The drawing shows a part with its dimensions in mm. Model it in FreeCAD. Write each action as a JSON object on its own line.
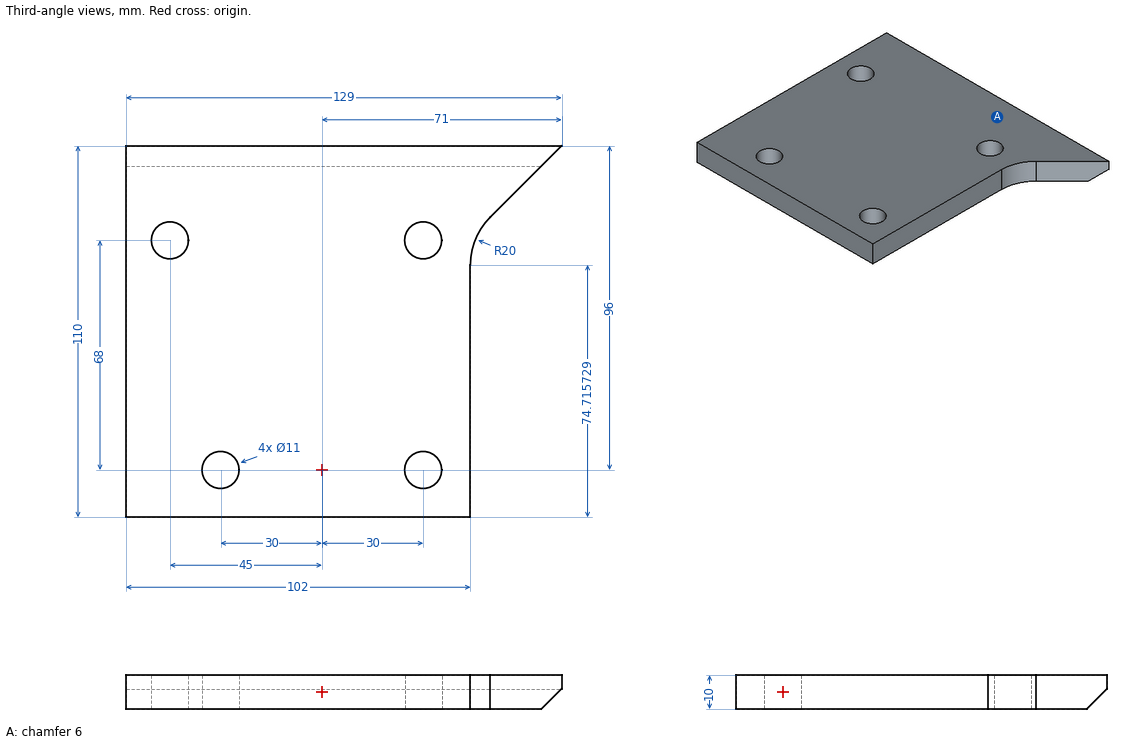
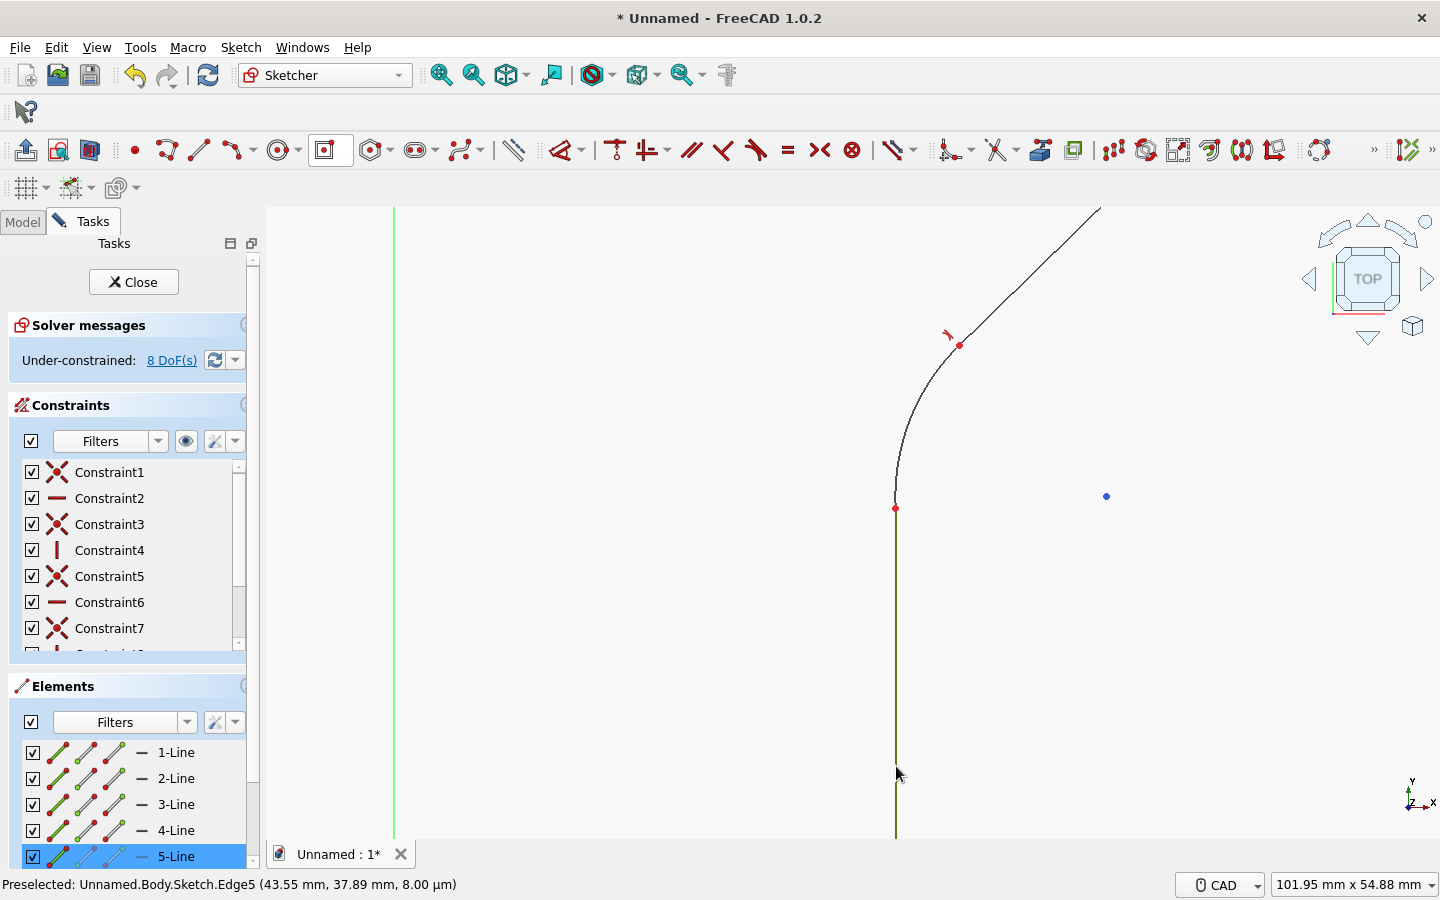
{"action": "left_click", "coordinate": [926, 388]}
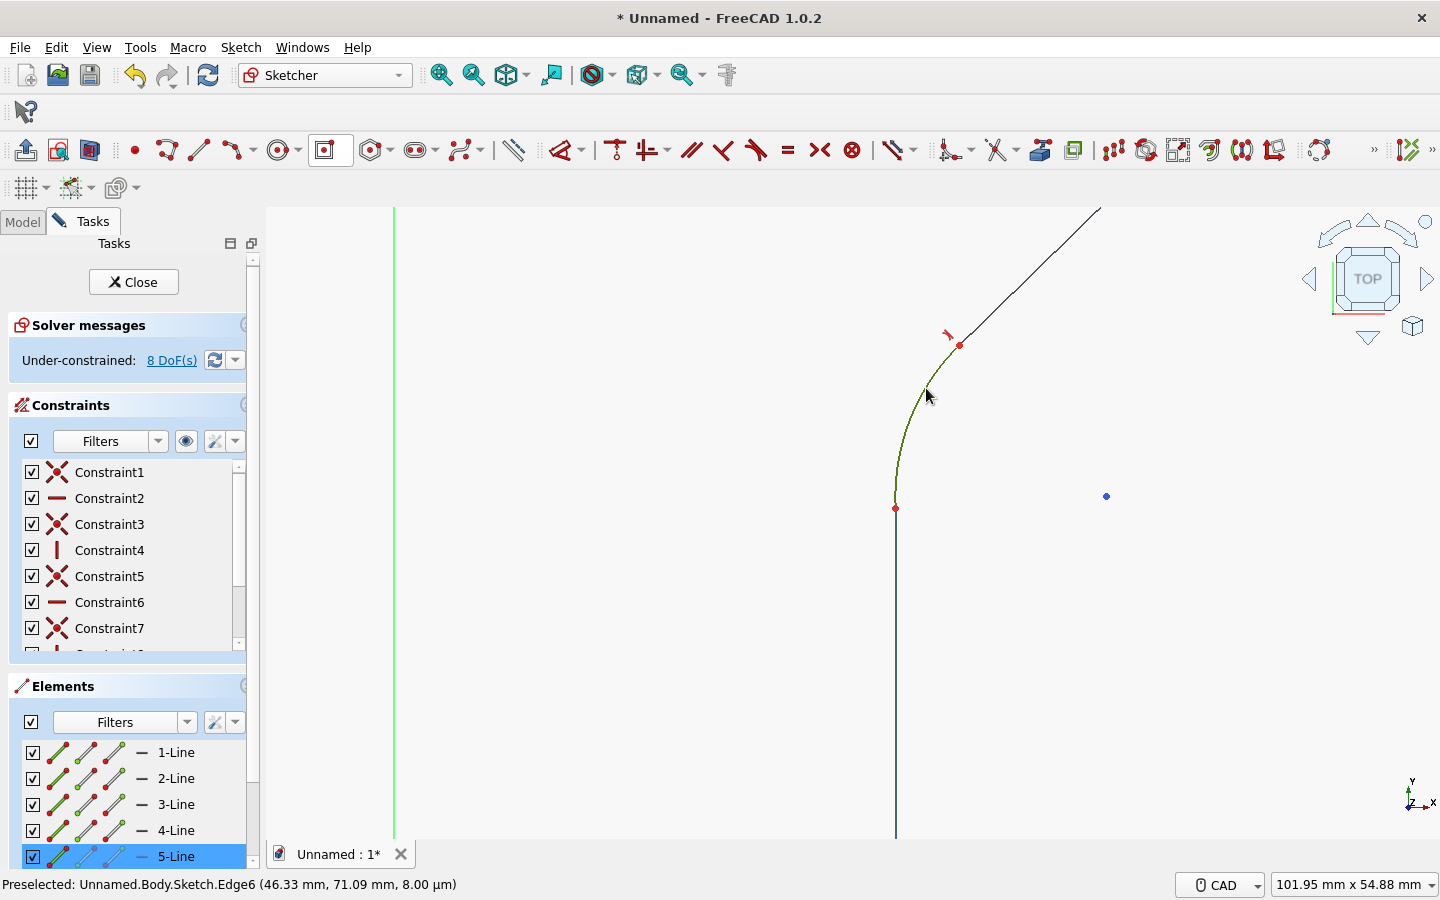
{"action": "left_click", "coordinate": [756, 150]}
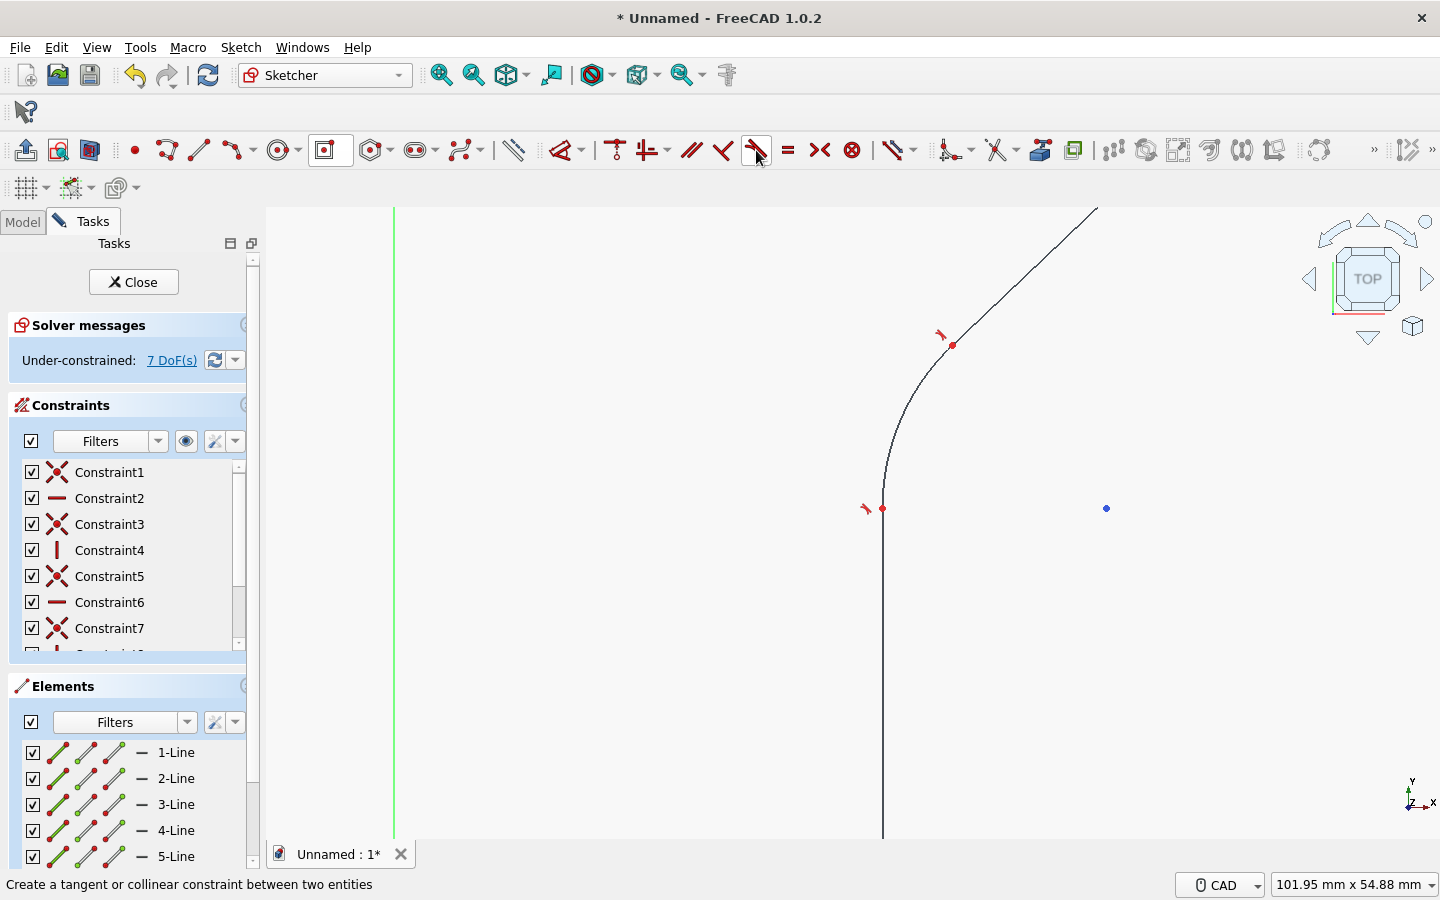
{"action": "key", "text": "d"}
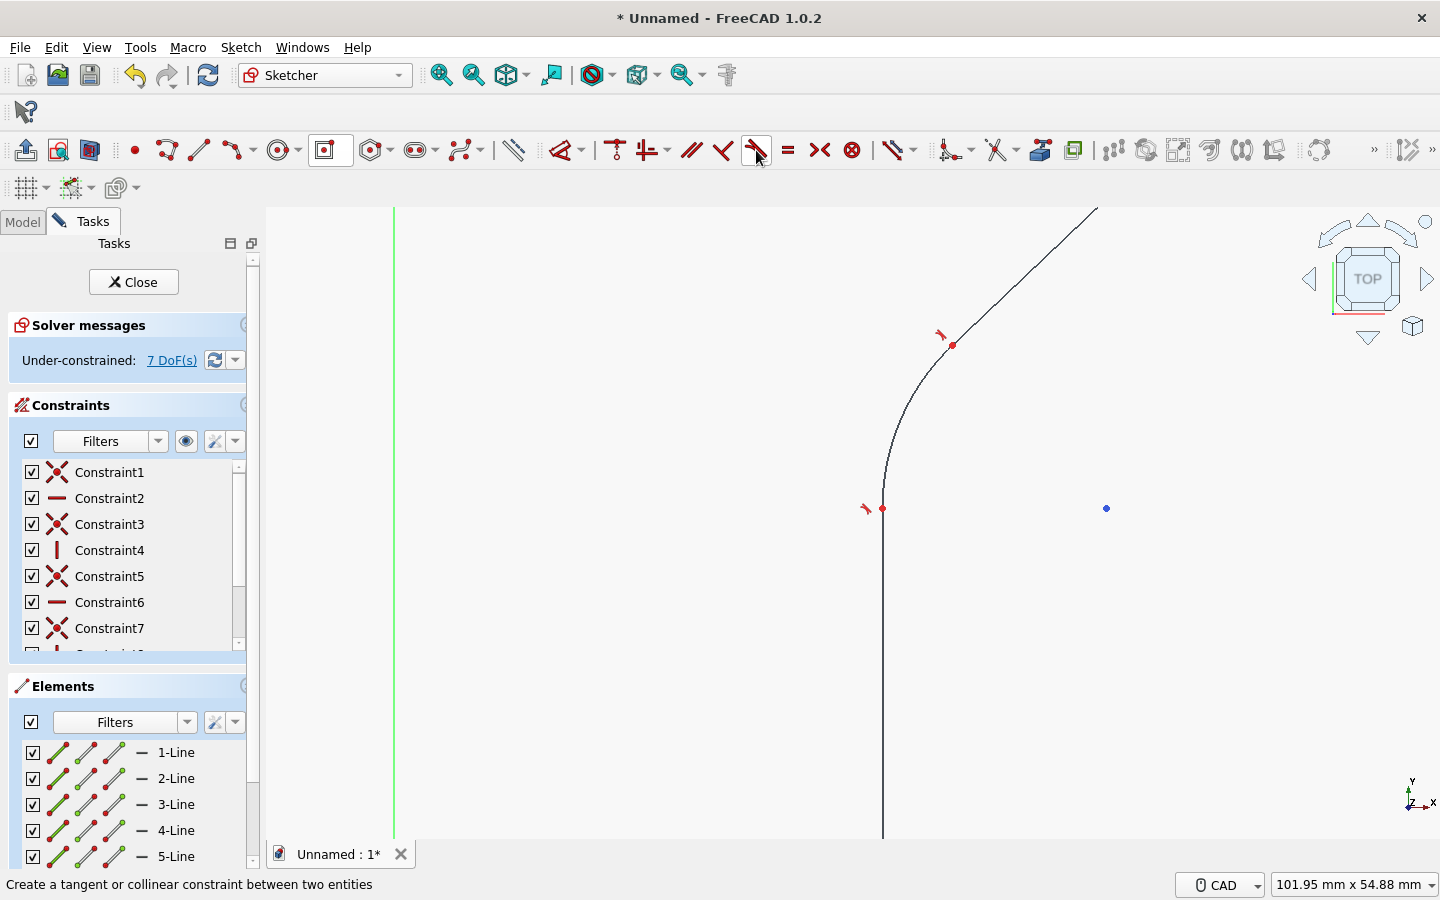
{"action": "left_click", "coordinate": [918, 388]}
{"action": "left_click", "coordinate": [891, 371]}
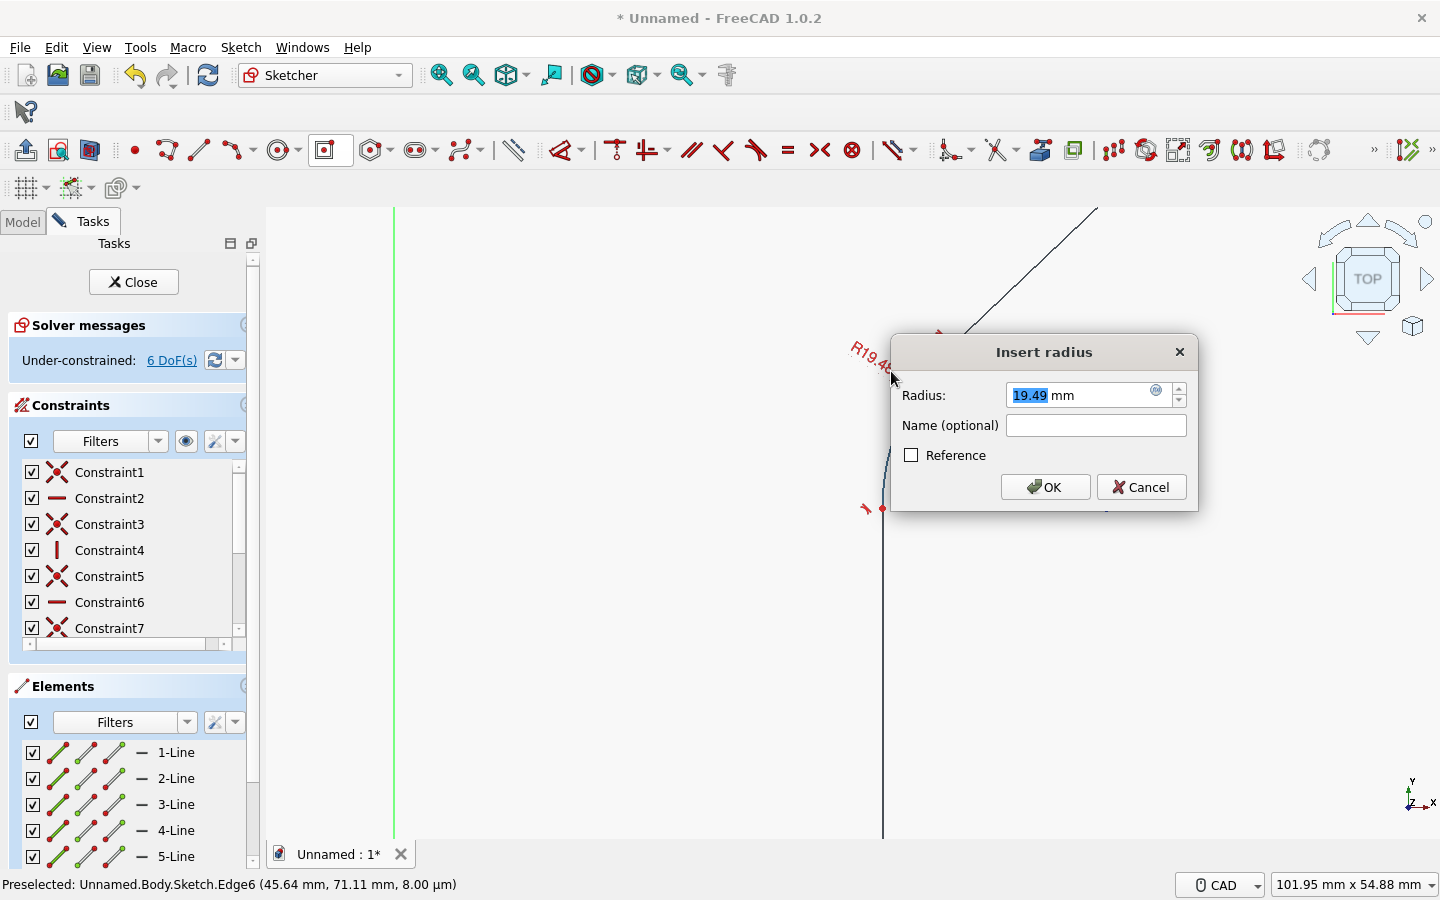
{"action": "type", "text": "20"}
{"action": "key", "text": "Return"}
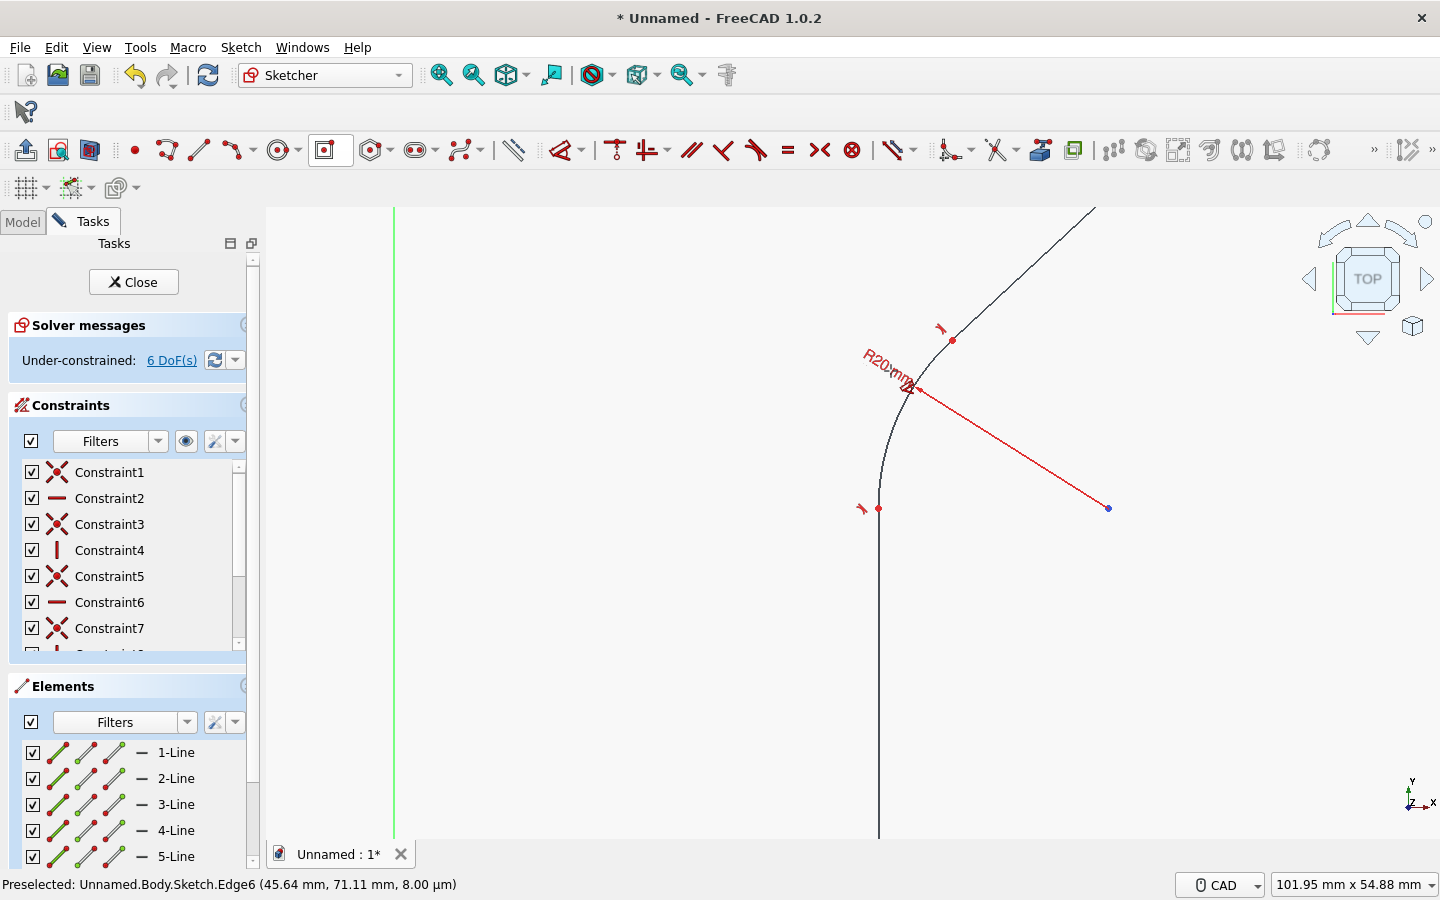
{"action": "scroll", "coordinate": [920, 433], "scroll_direction": "down", "scroll_amount": 6}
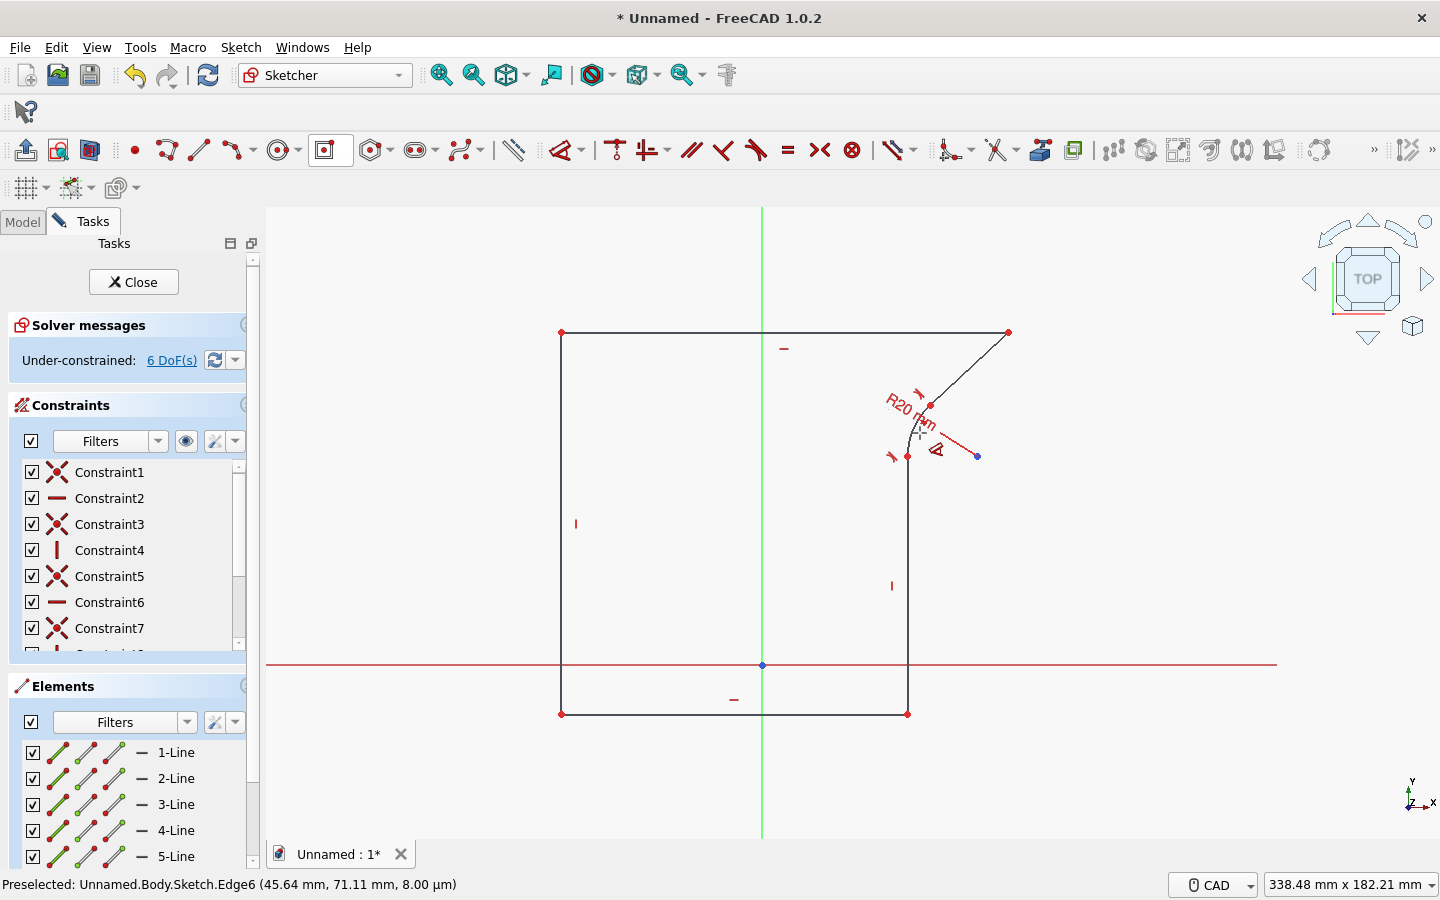
{"action": "left_click", "coordinate": [874, 333]}
{"action": "left_click", "coordinate": [785, 299]}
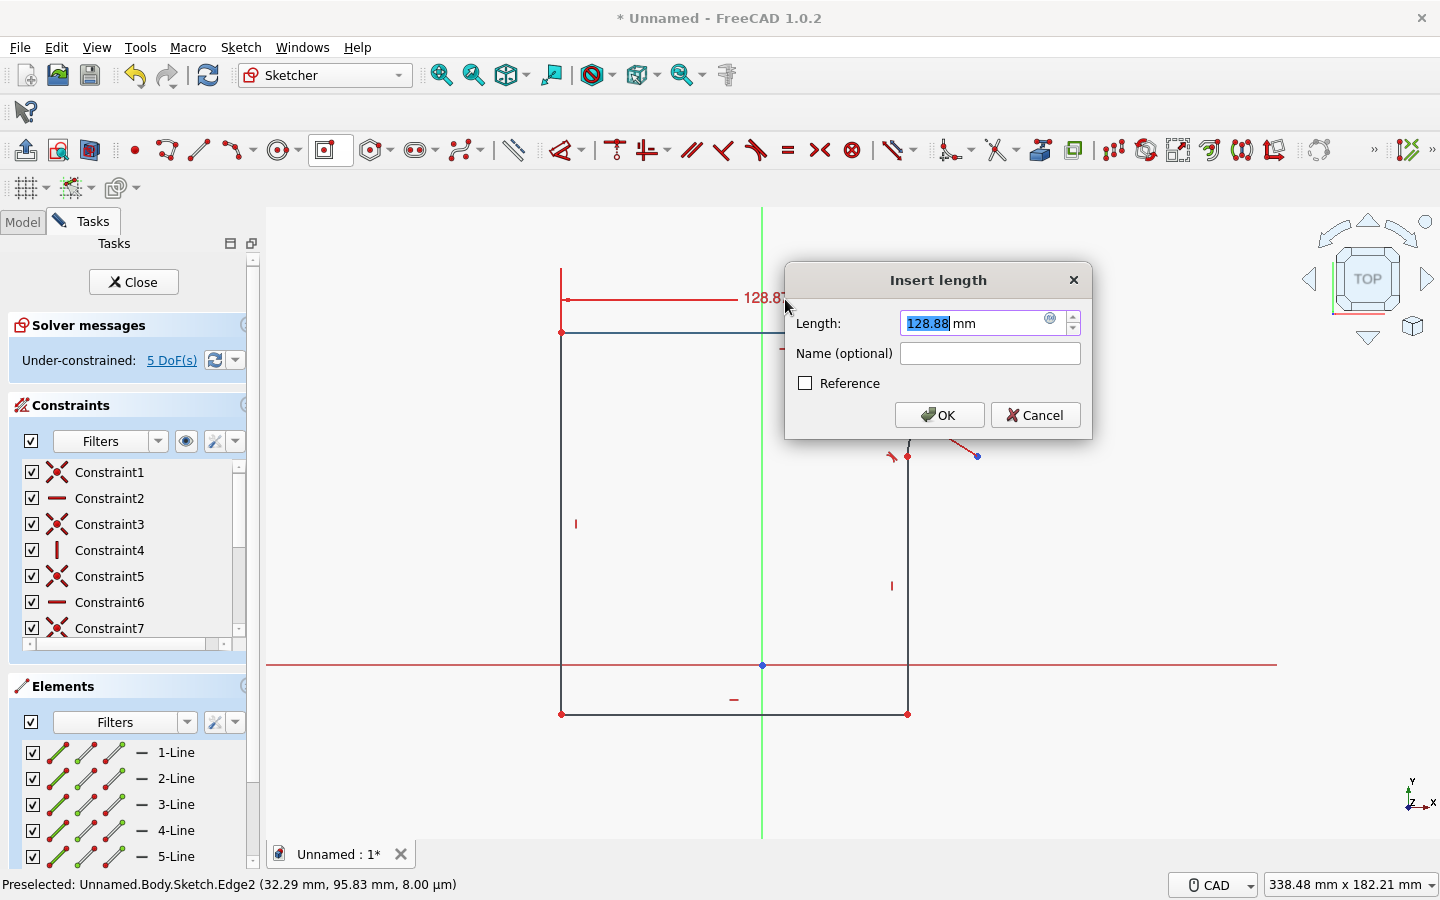
{"action": "type", "text": "129"}
{"action": "key", "text": "Return"}